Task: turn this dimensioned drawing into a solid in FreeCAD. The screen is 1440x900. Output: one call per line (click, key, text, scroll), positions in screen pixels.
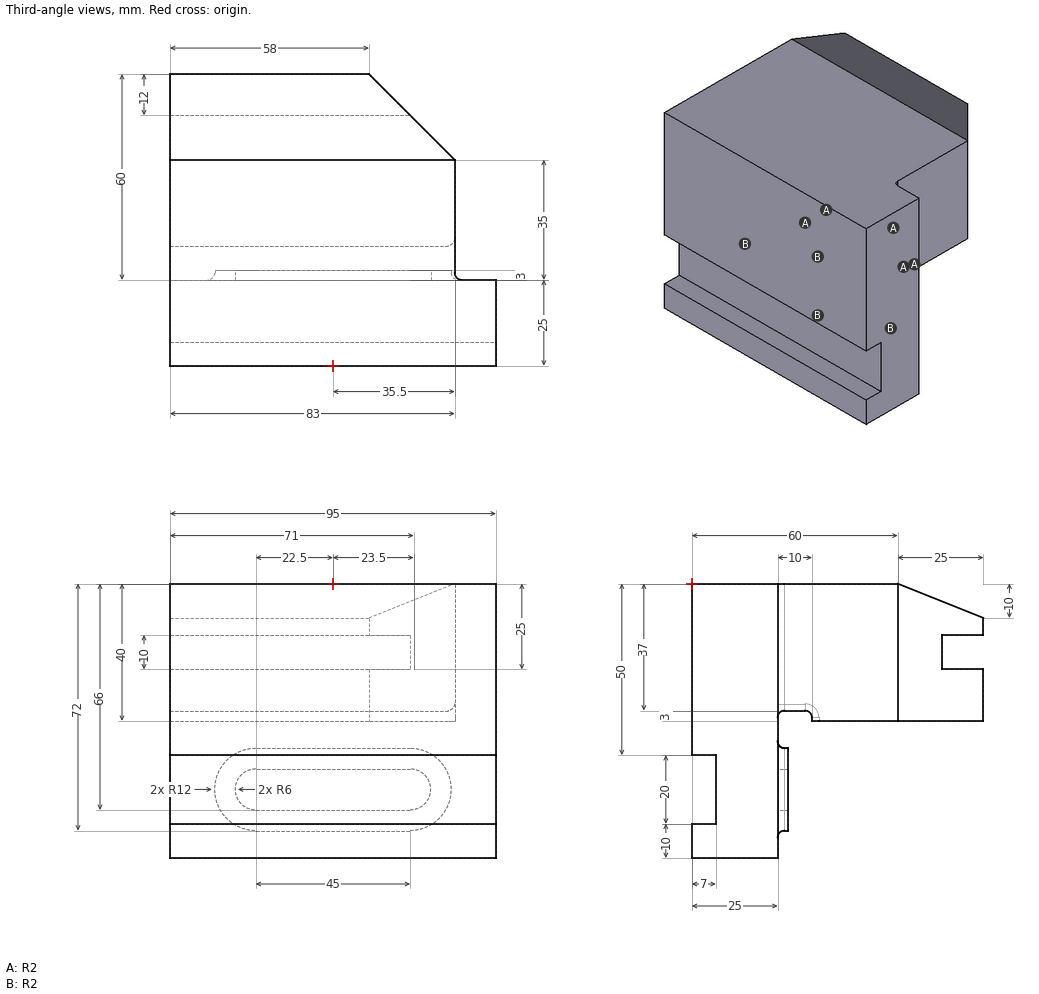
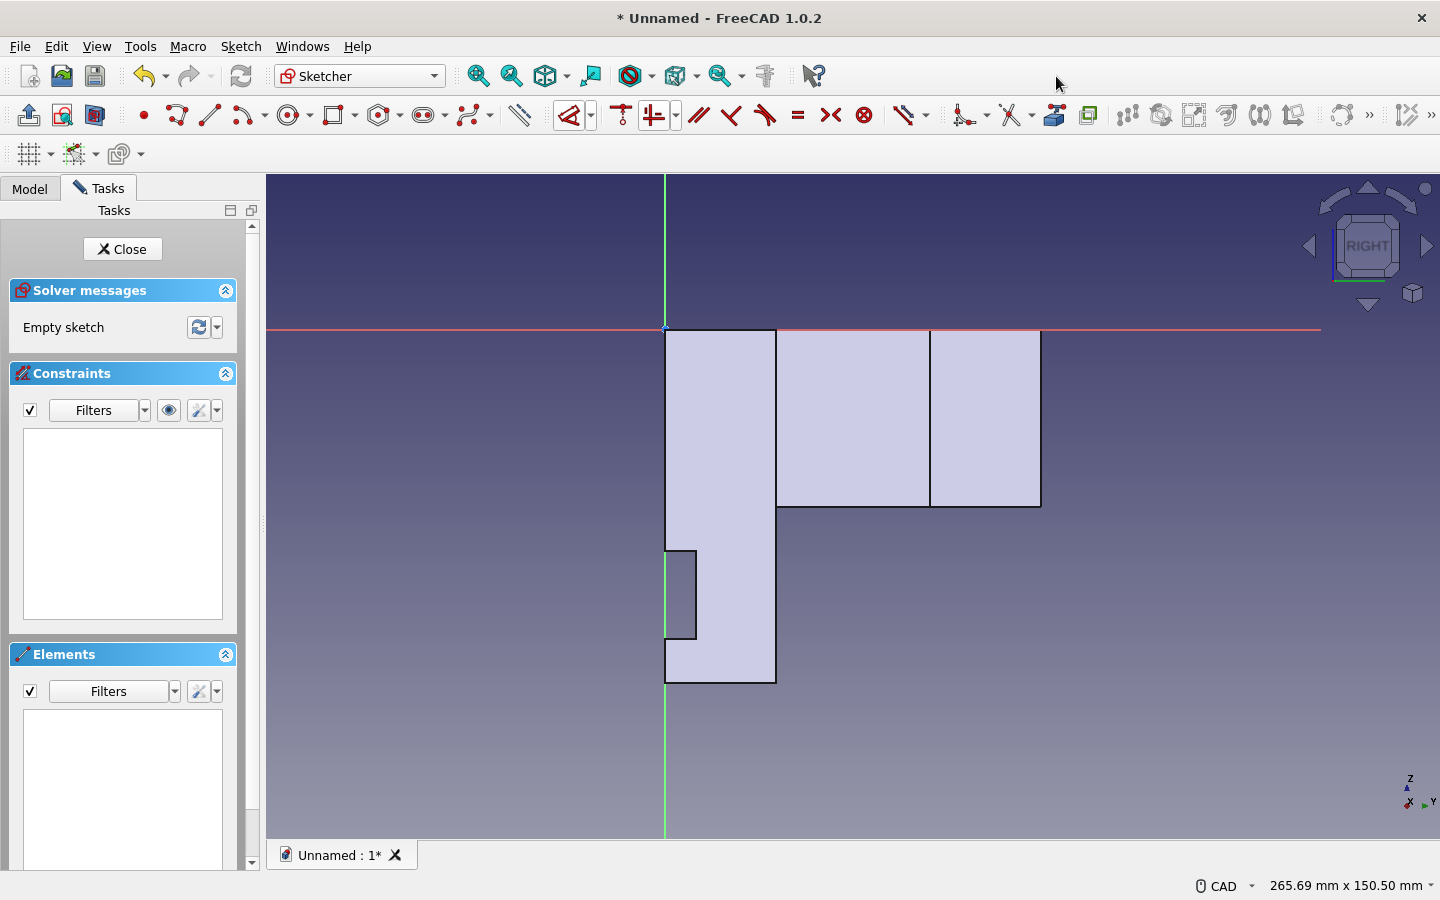
scroll(799, 499, up, 14)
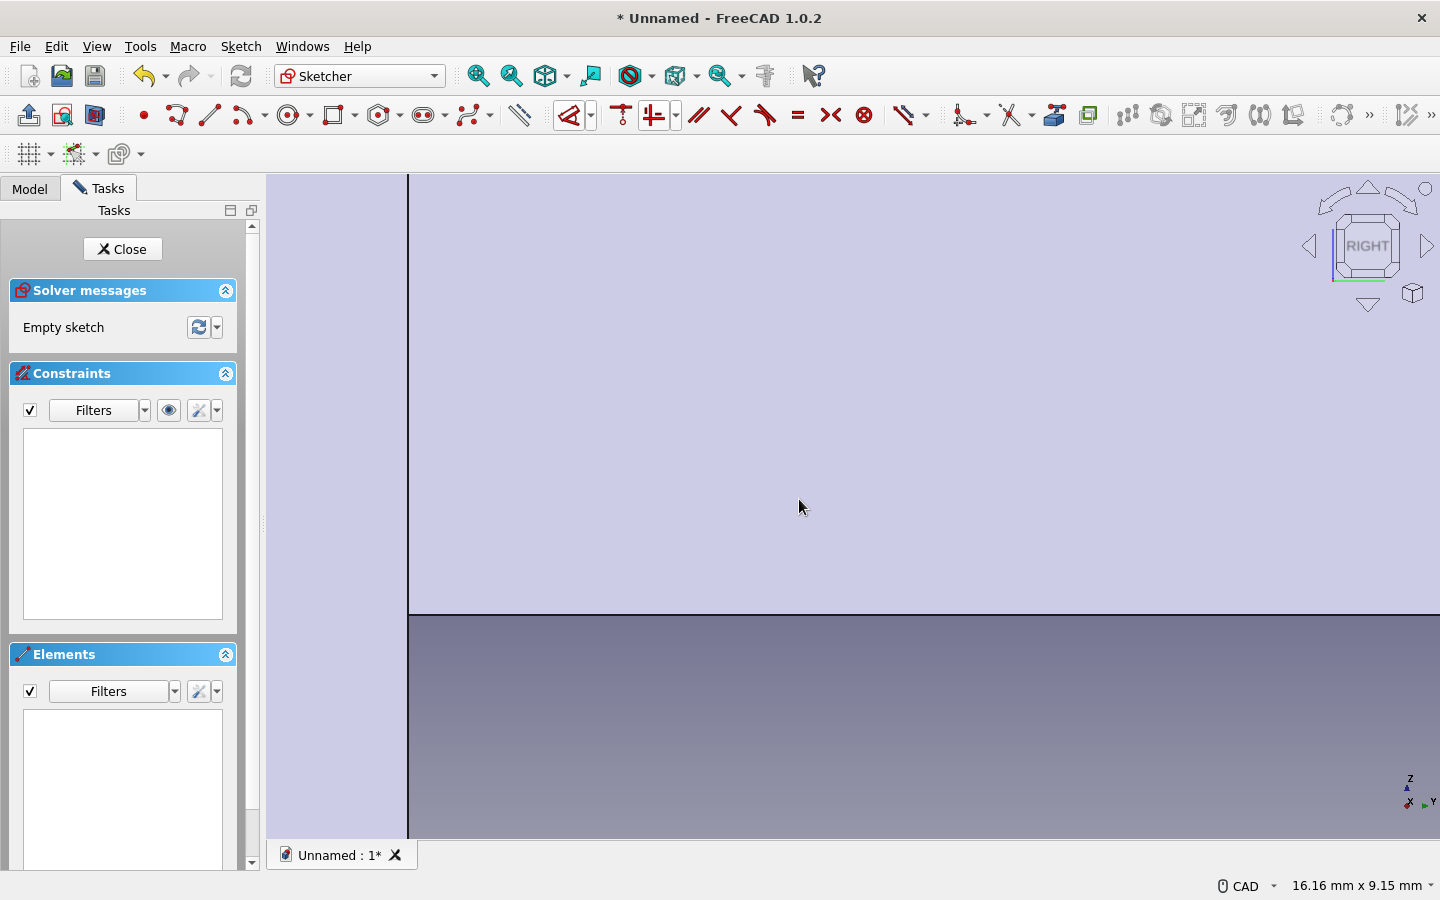
click(332, 116)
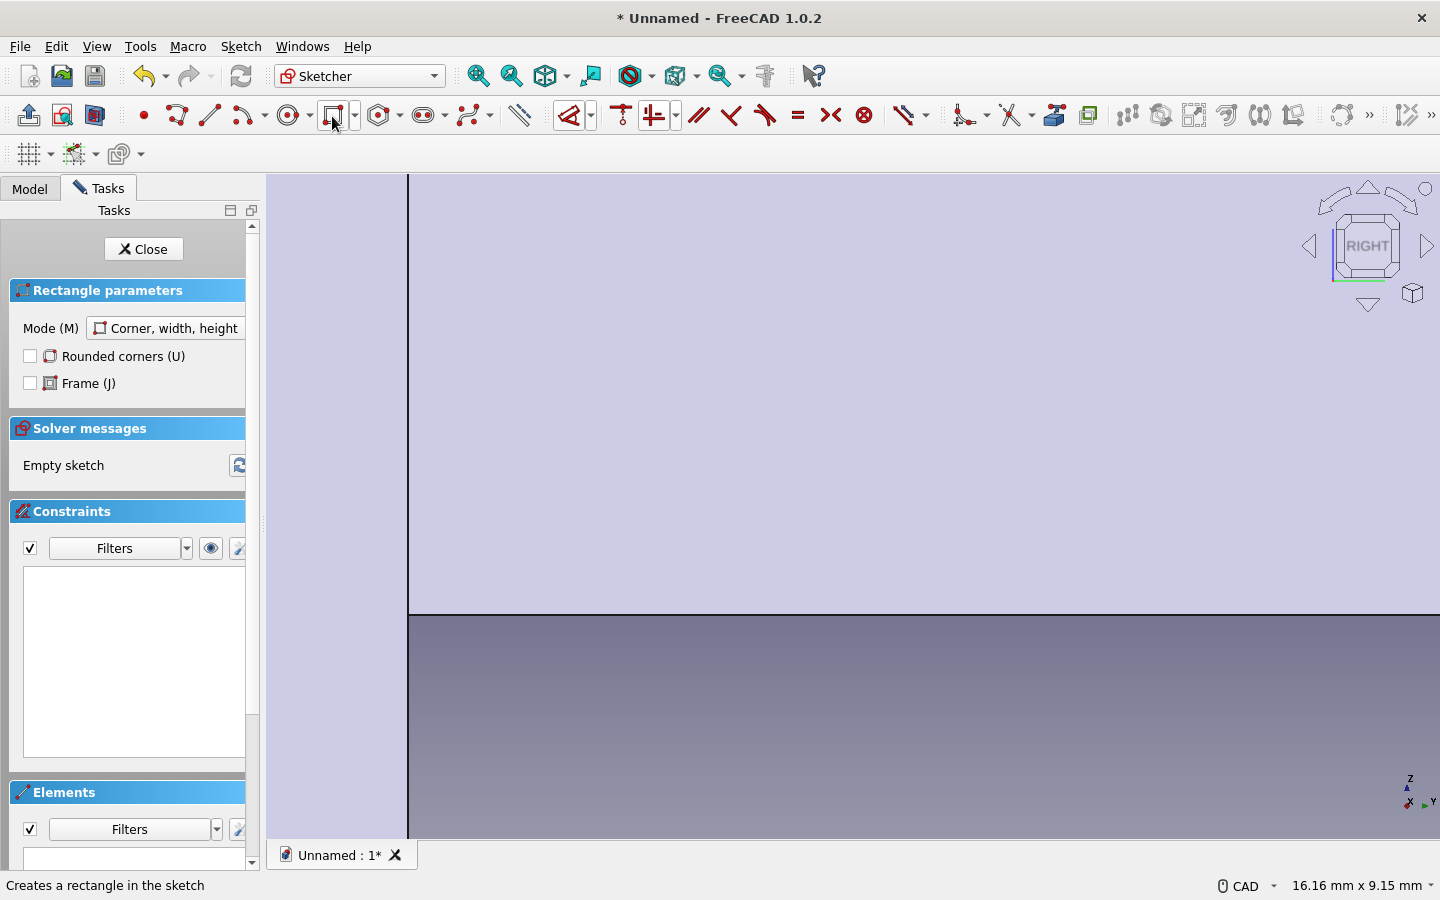
click(408, 397)
click(1135, 615)
key(Escape)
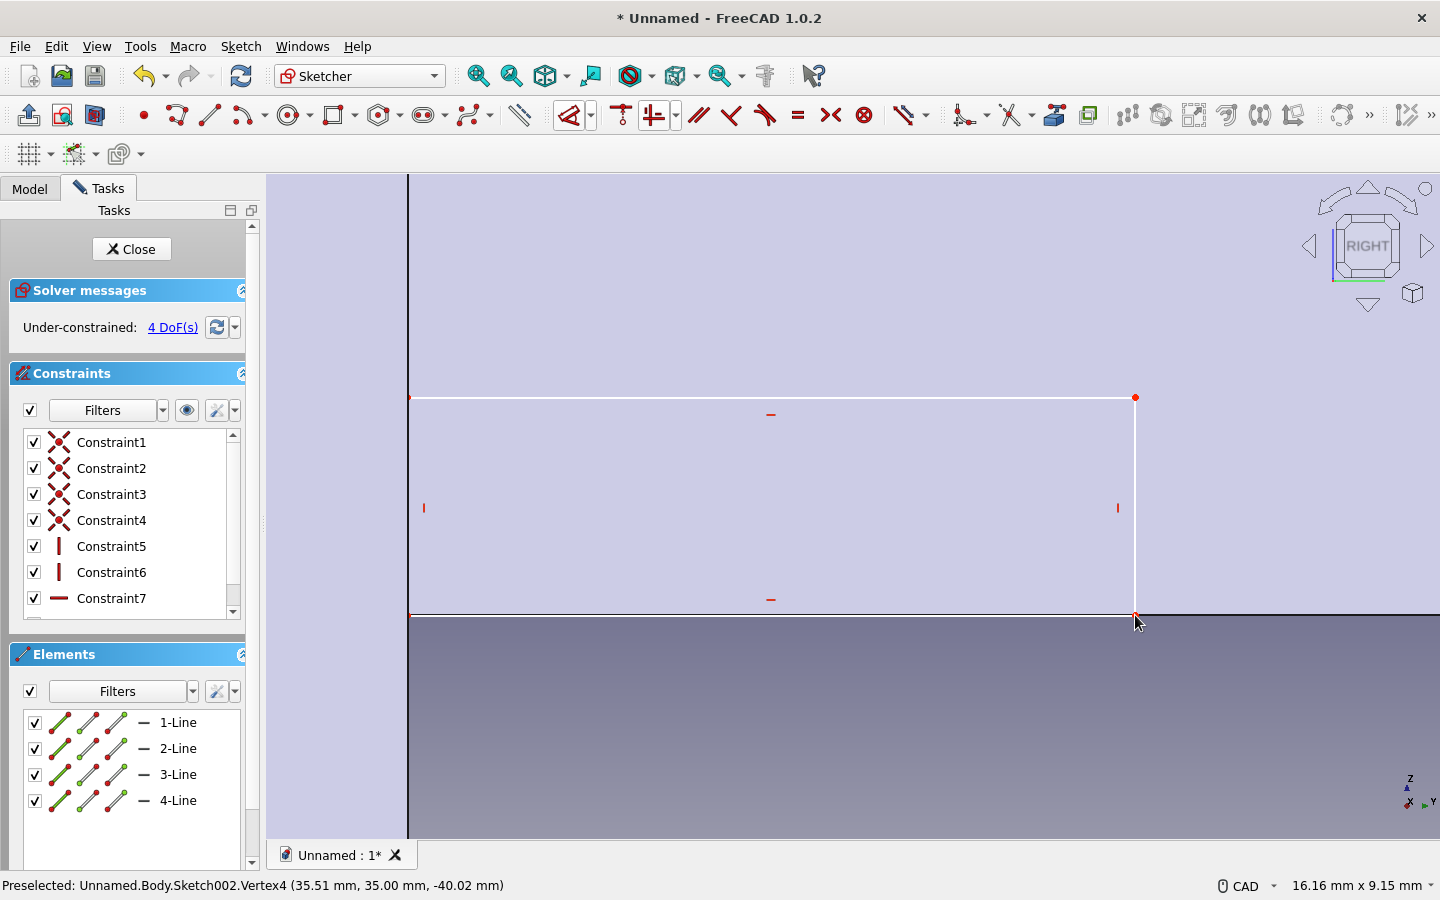
click(408, 463)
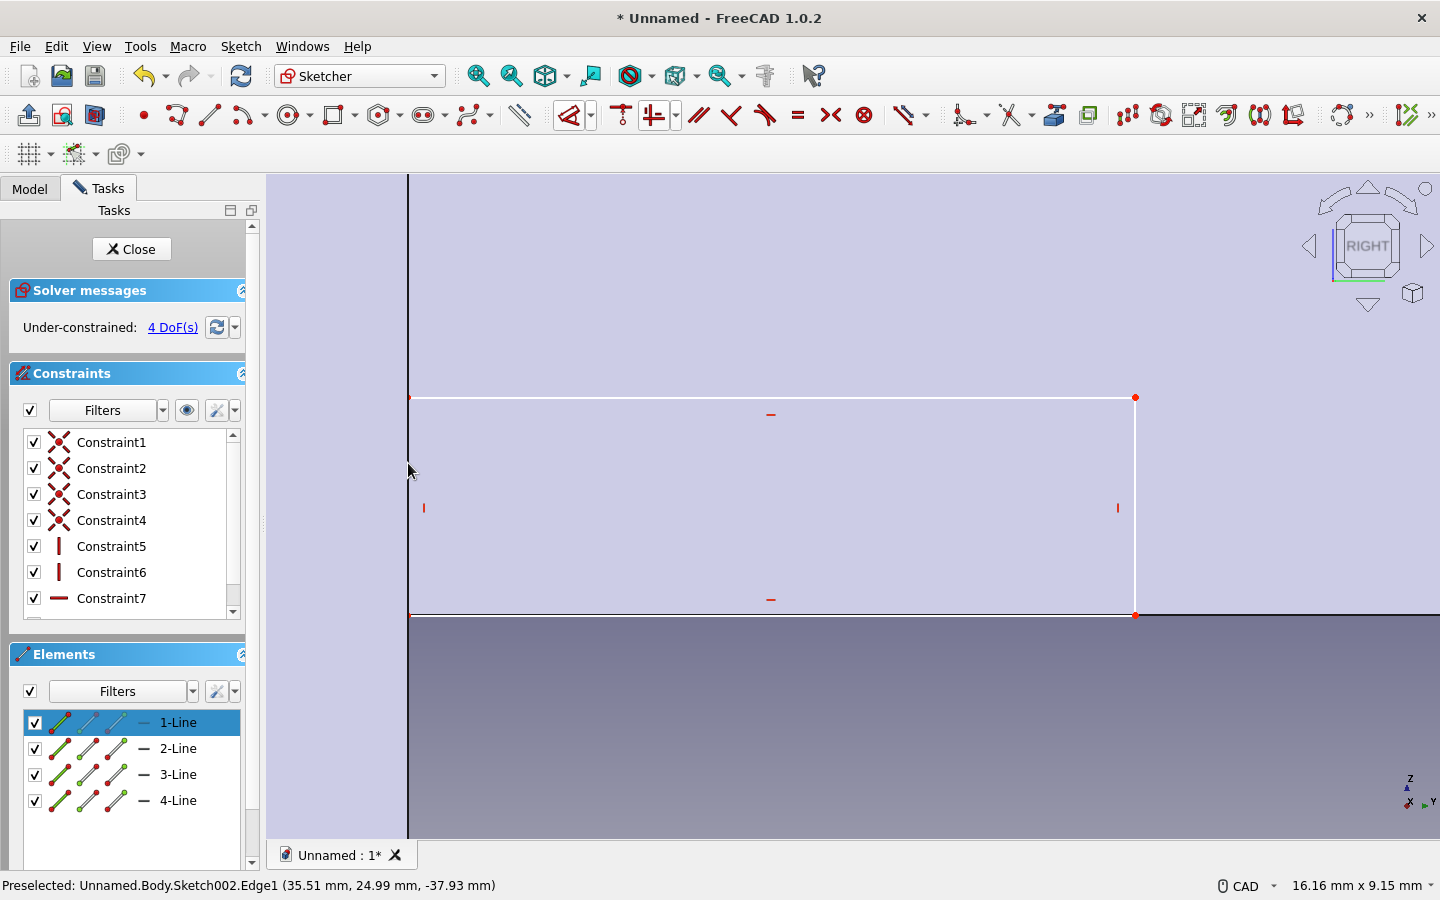
click(590, 116)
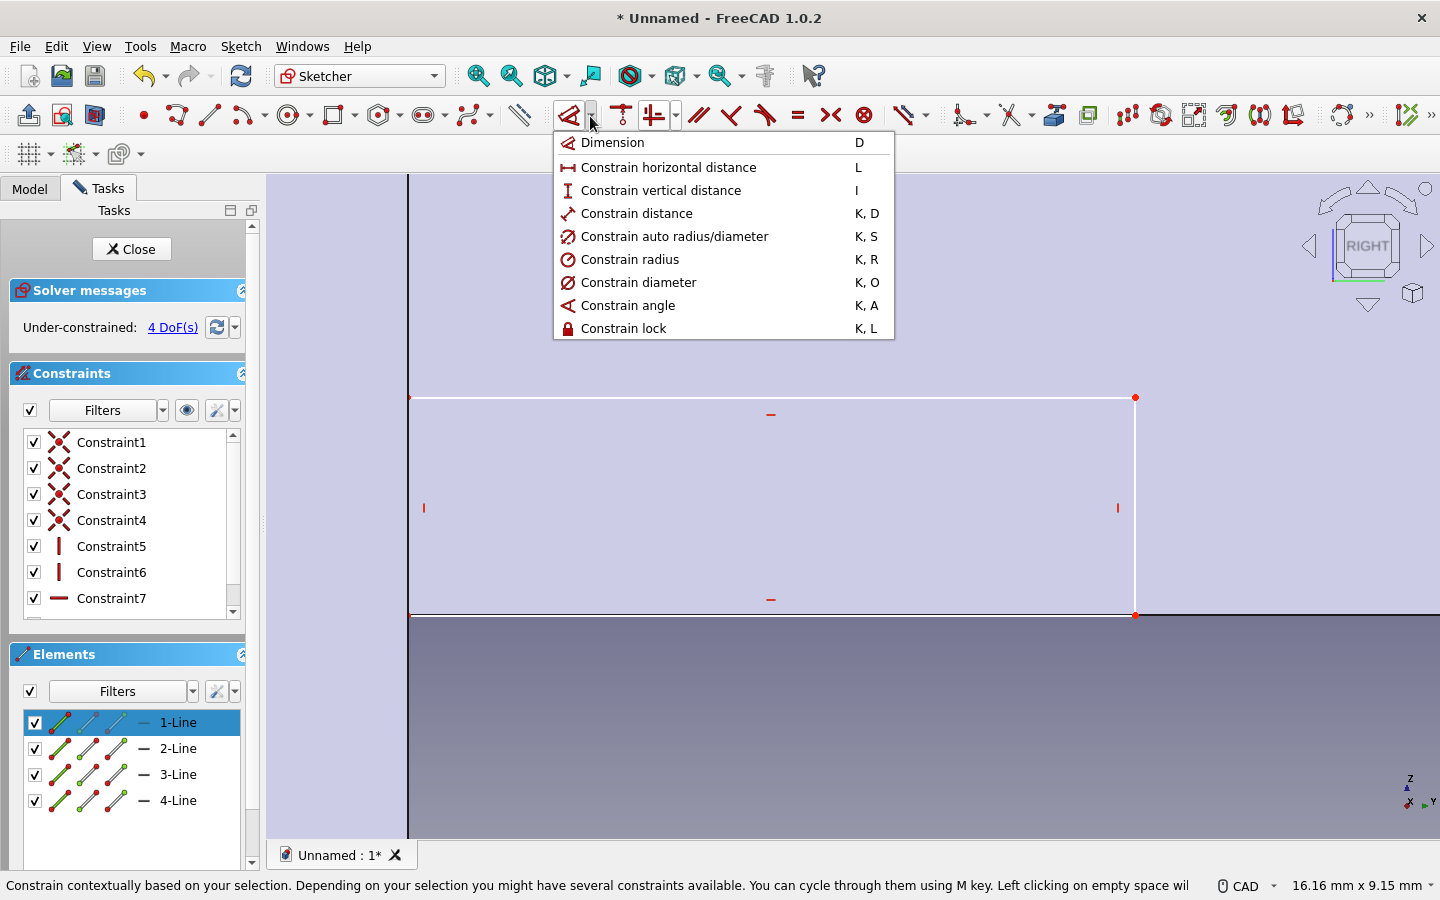
click(724, 190)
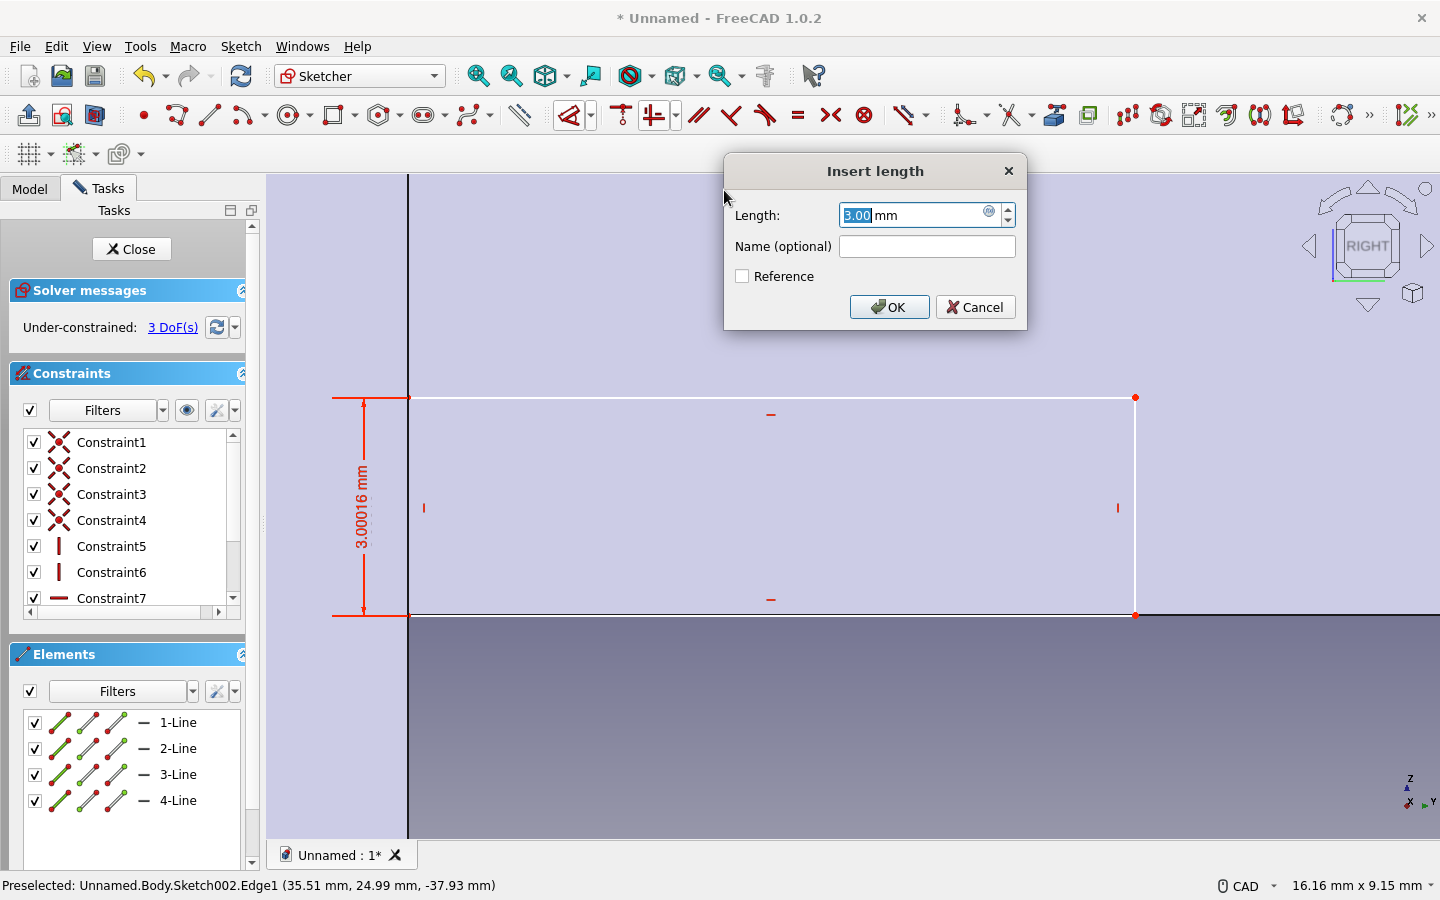
text(3)
key(Return)